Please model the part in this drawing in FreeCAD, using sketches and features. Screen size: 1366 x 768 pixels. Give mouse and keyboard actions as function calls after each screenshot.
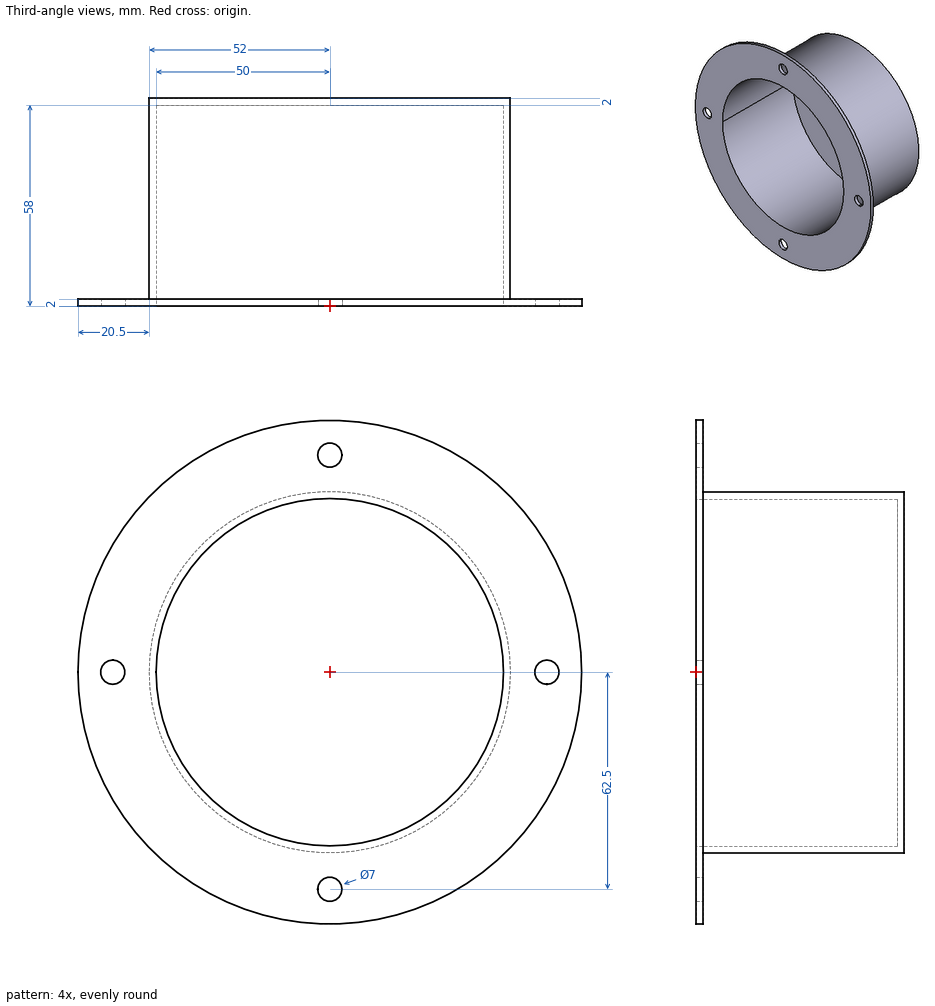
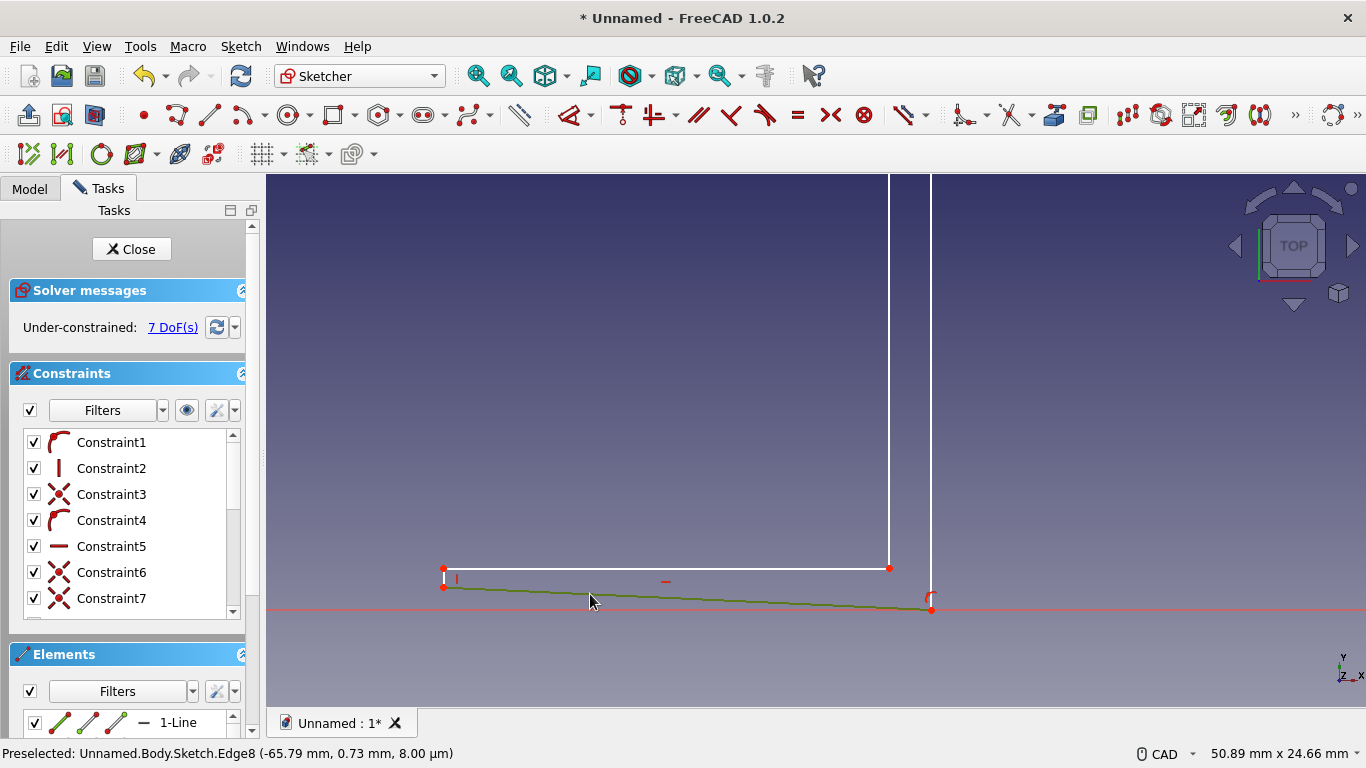
key(h)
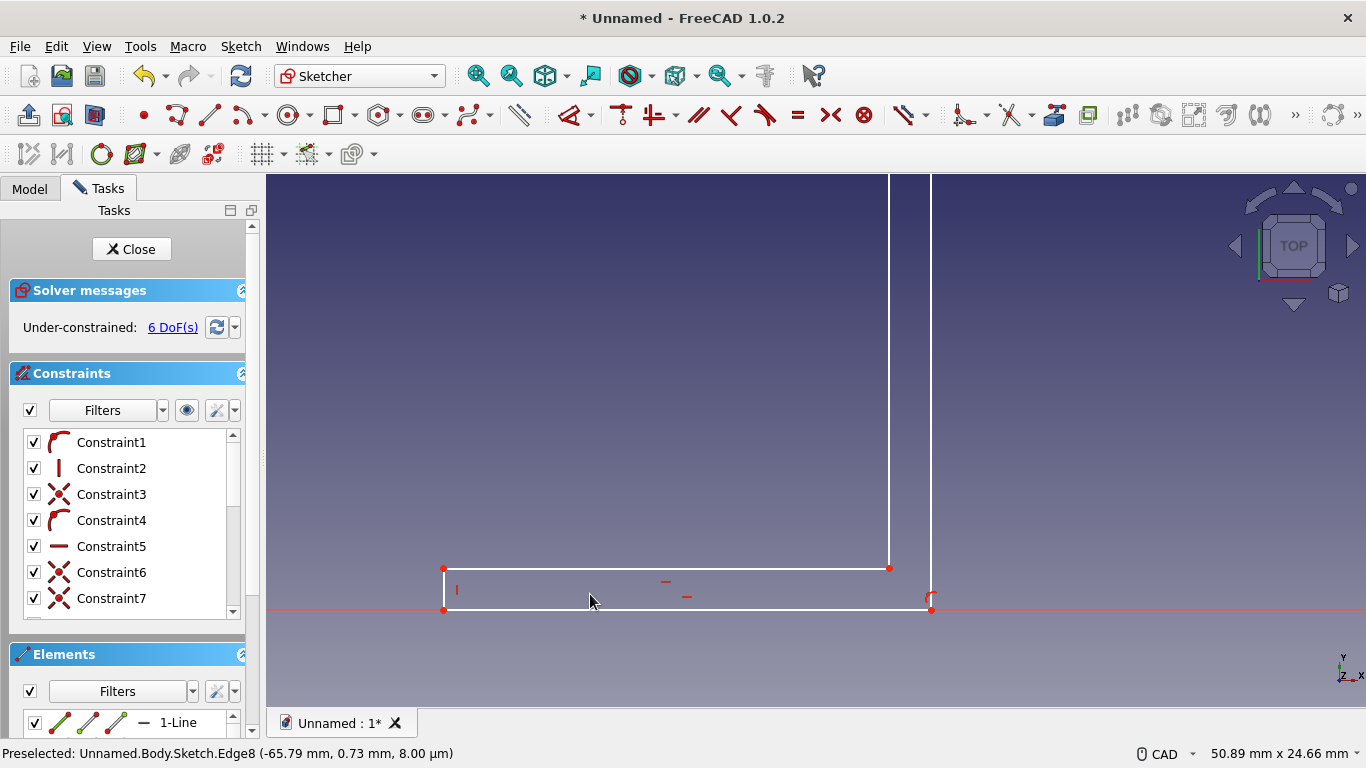
key(d)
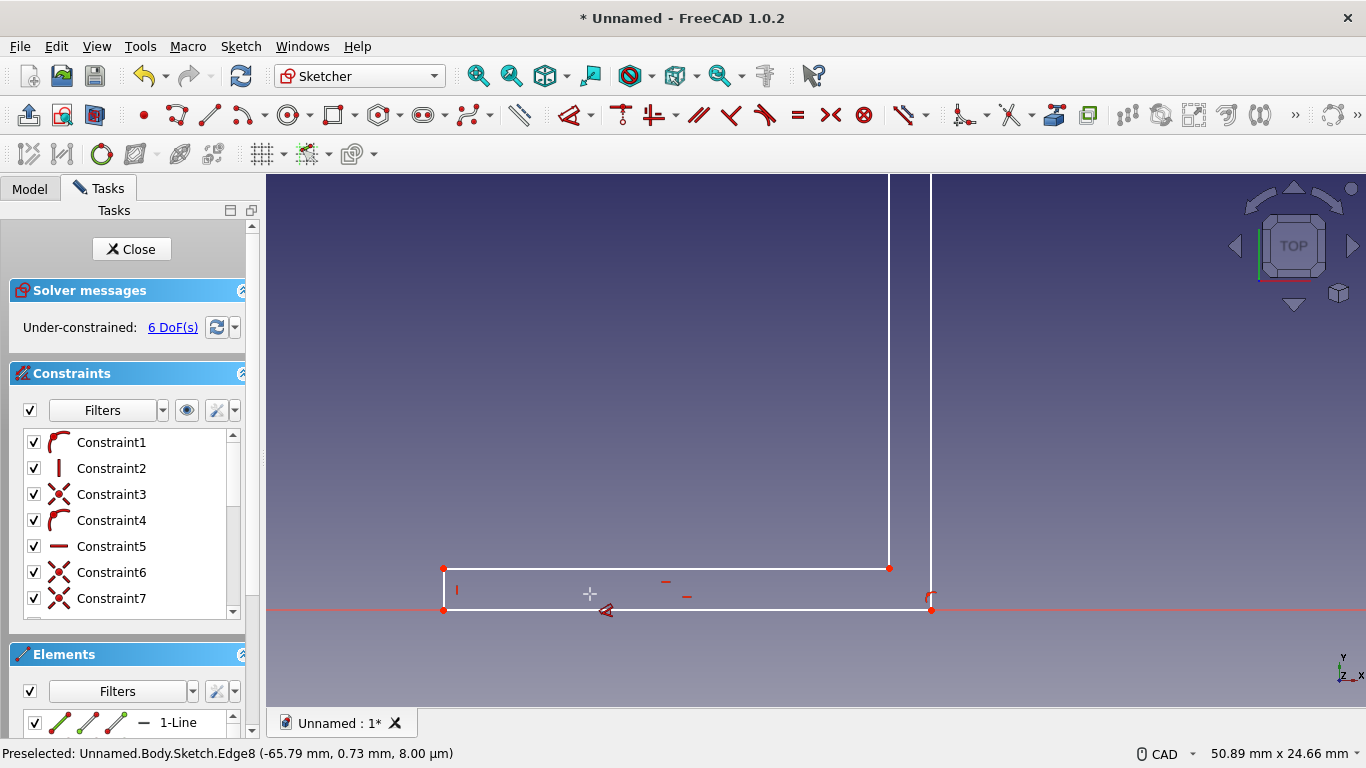
scroll(590, 597, down, 7)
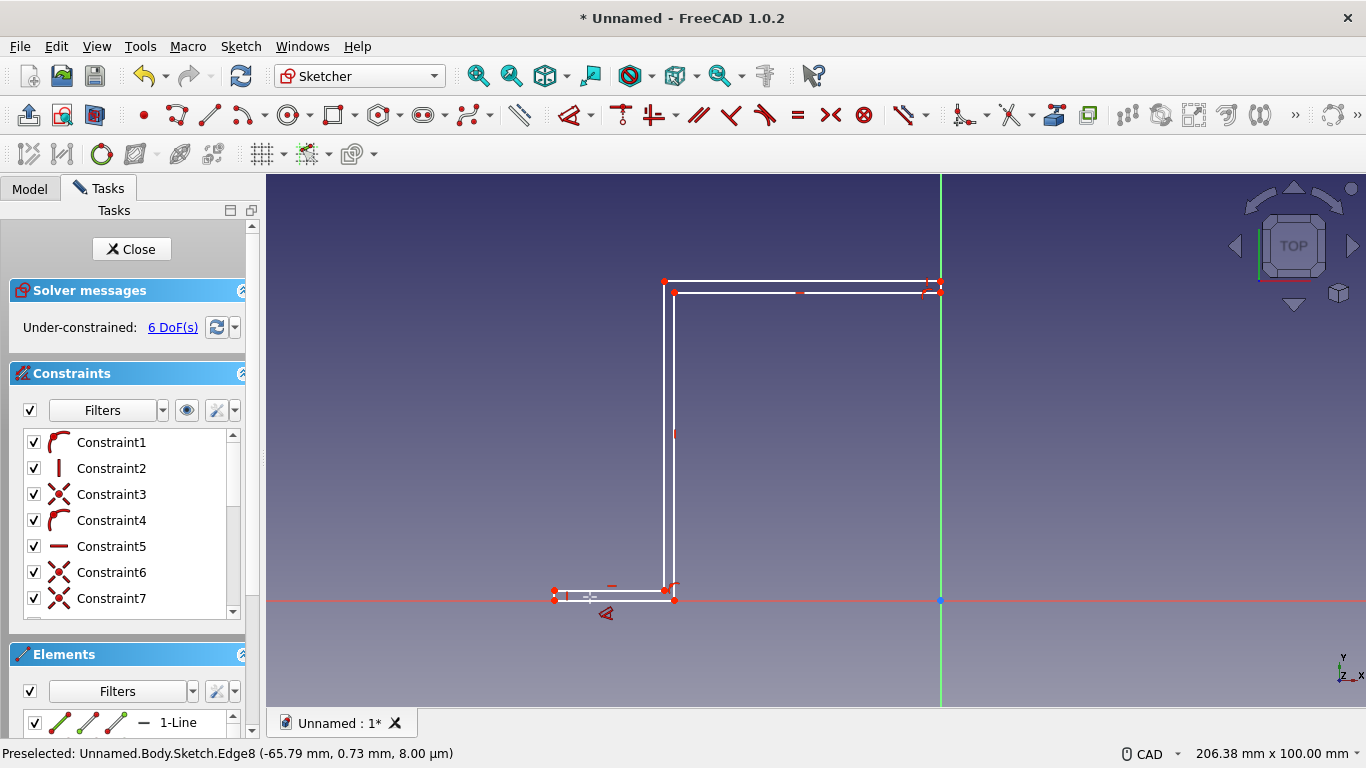
scroll(941, 289, up, 8)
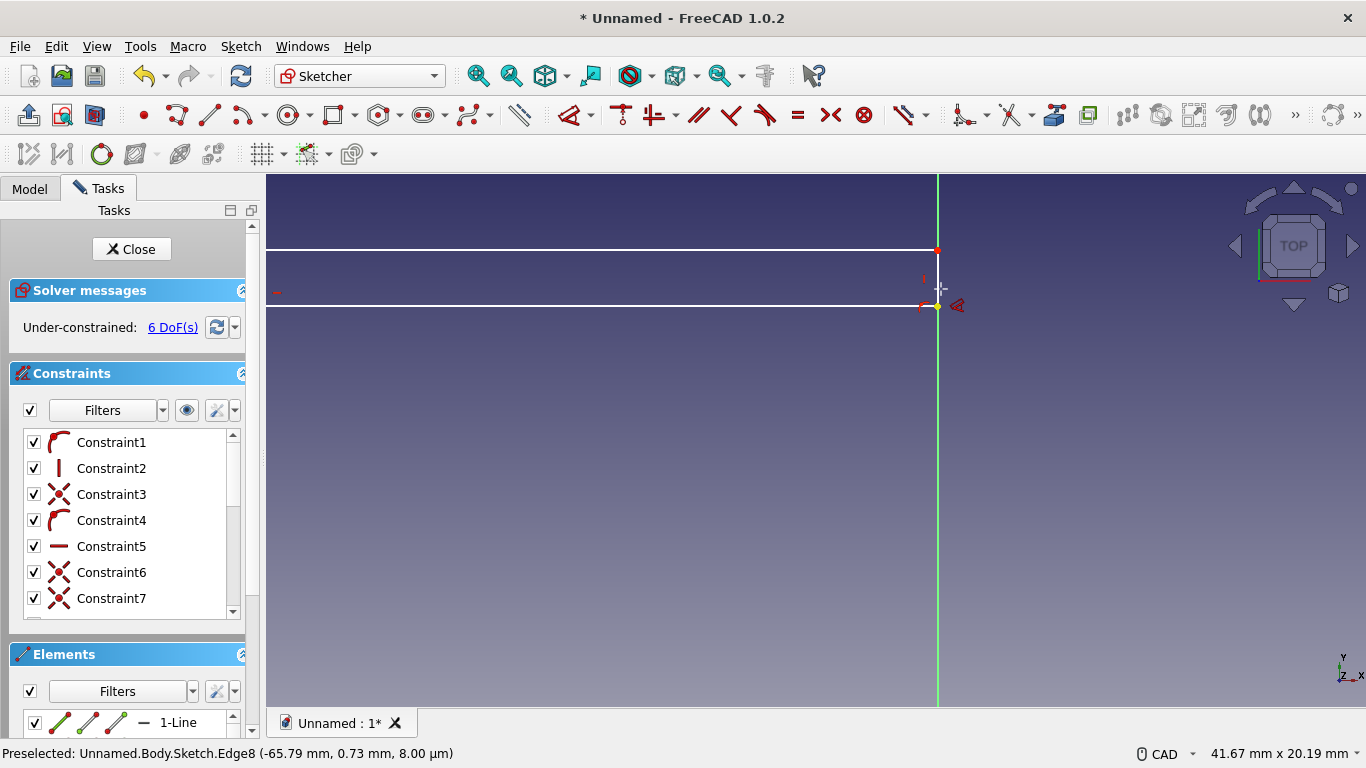
click(938, 290)
click(972, 278)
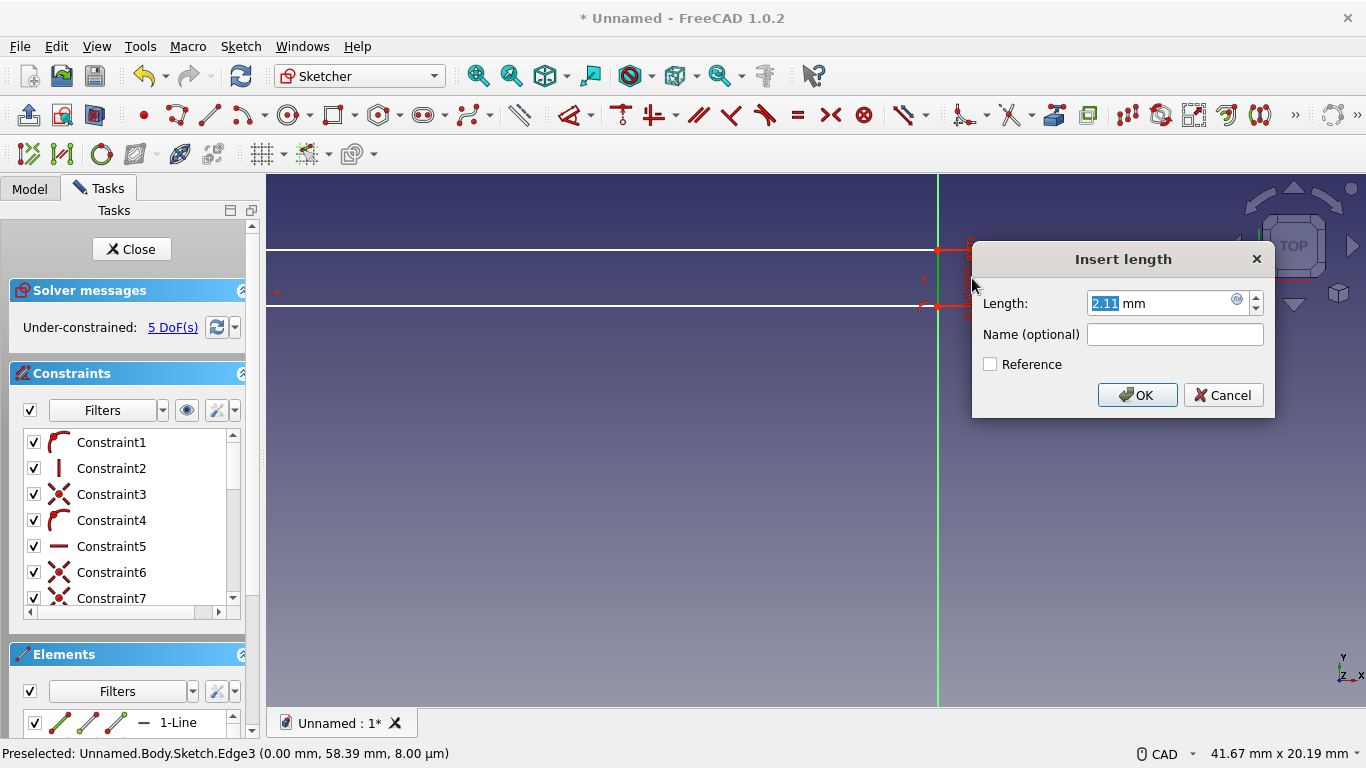
text(2)
key(Return)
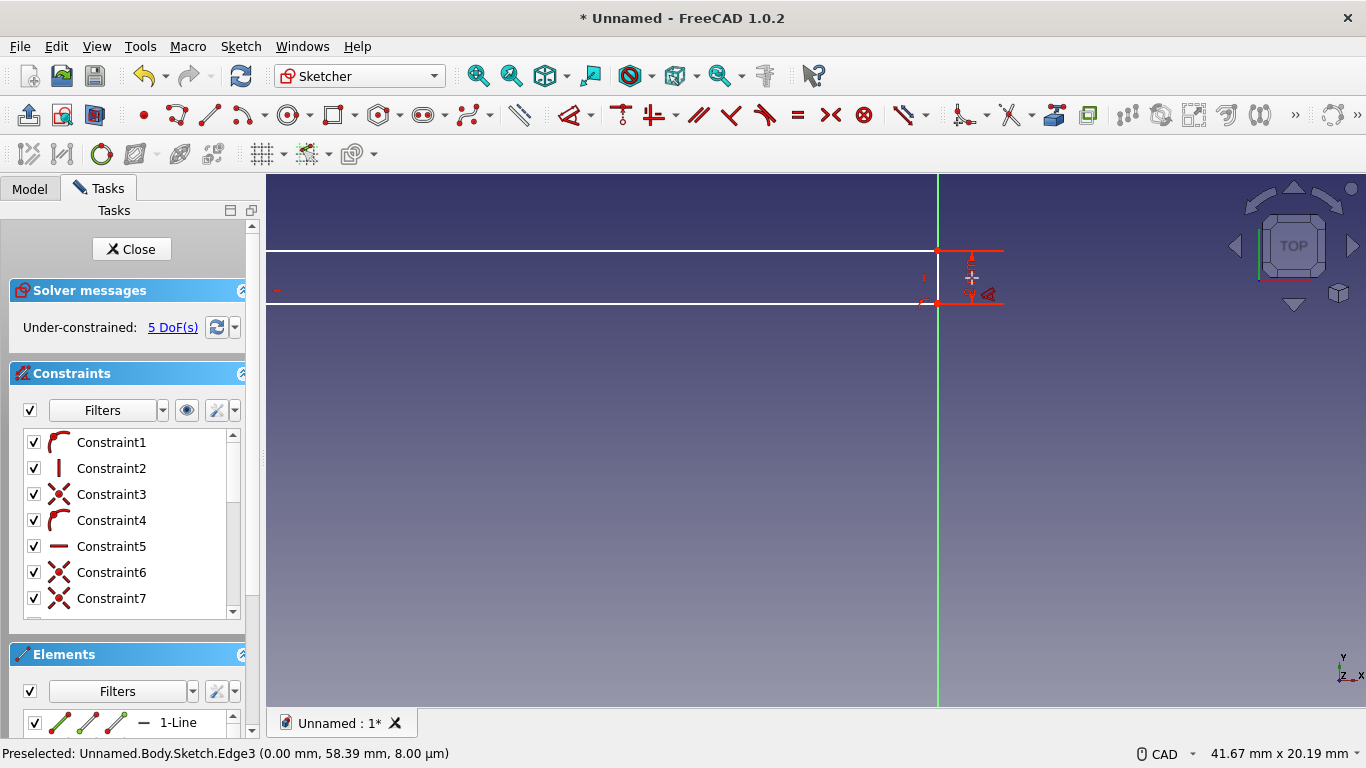
scroll(941, 289, down, 8)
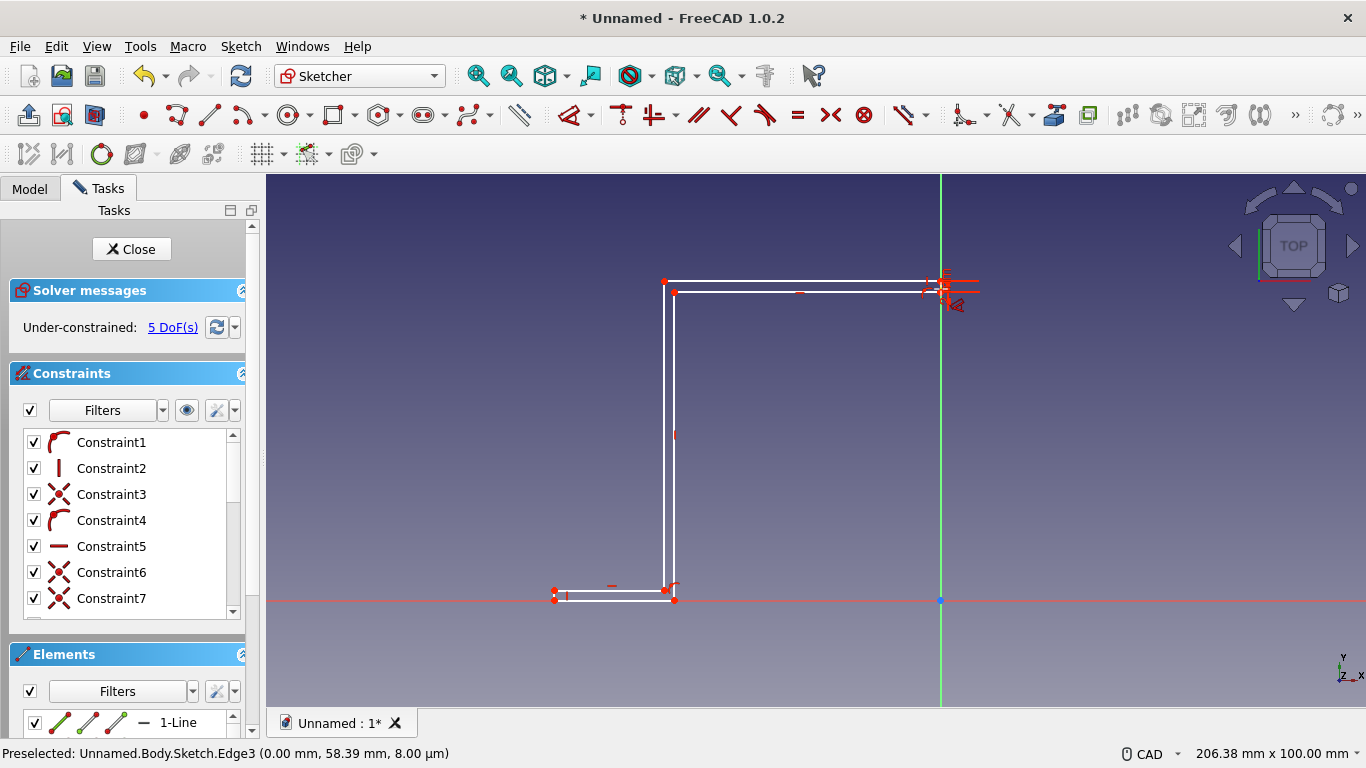
scroll(554, 594, up, 8)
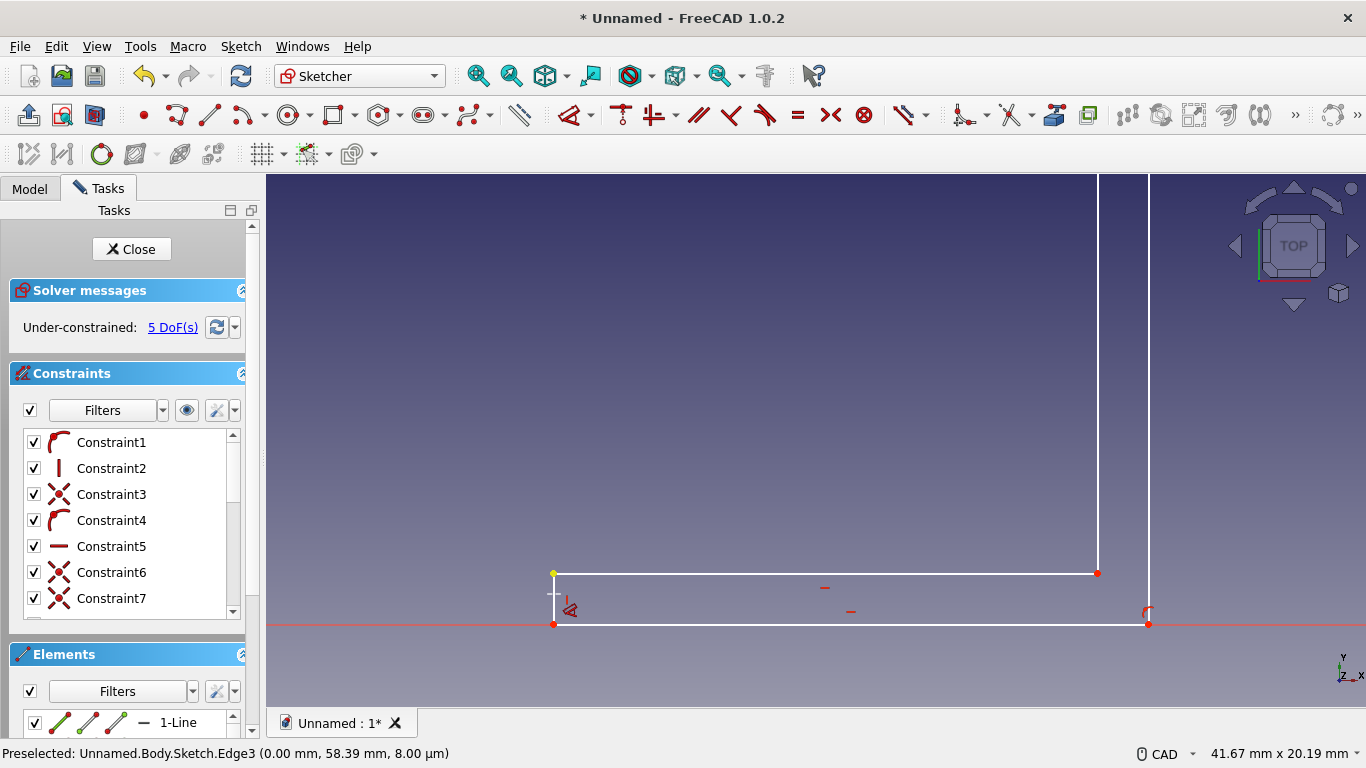
click(554, 589)
click(520, 599)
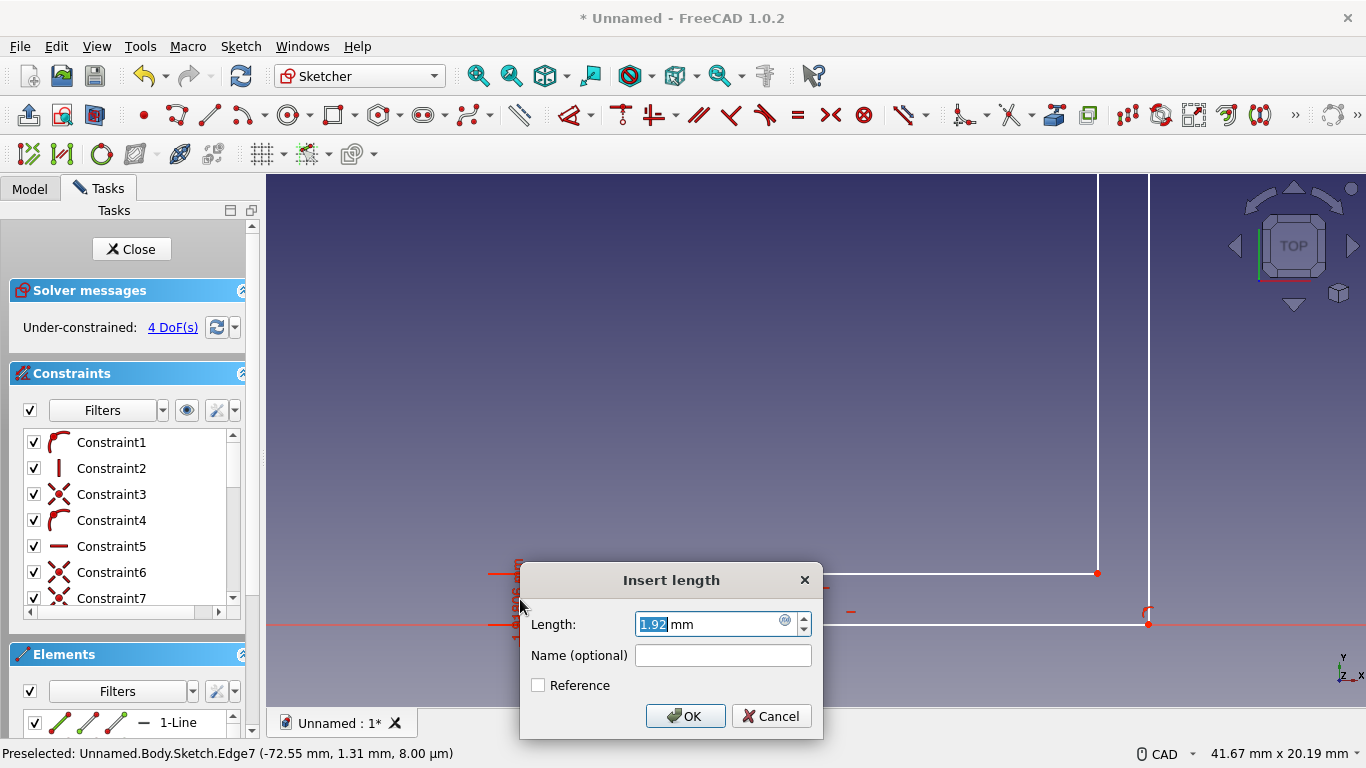
text(2)
key(Return)